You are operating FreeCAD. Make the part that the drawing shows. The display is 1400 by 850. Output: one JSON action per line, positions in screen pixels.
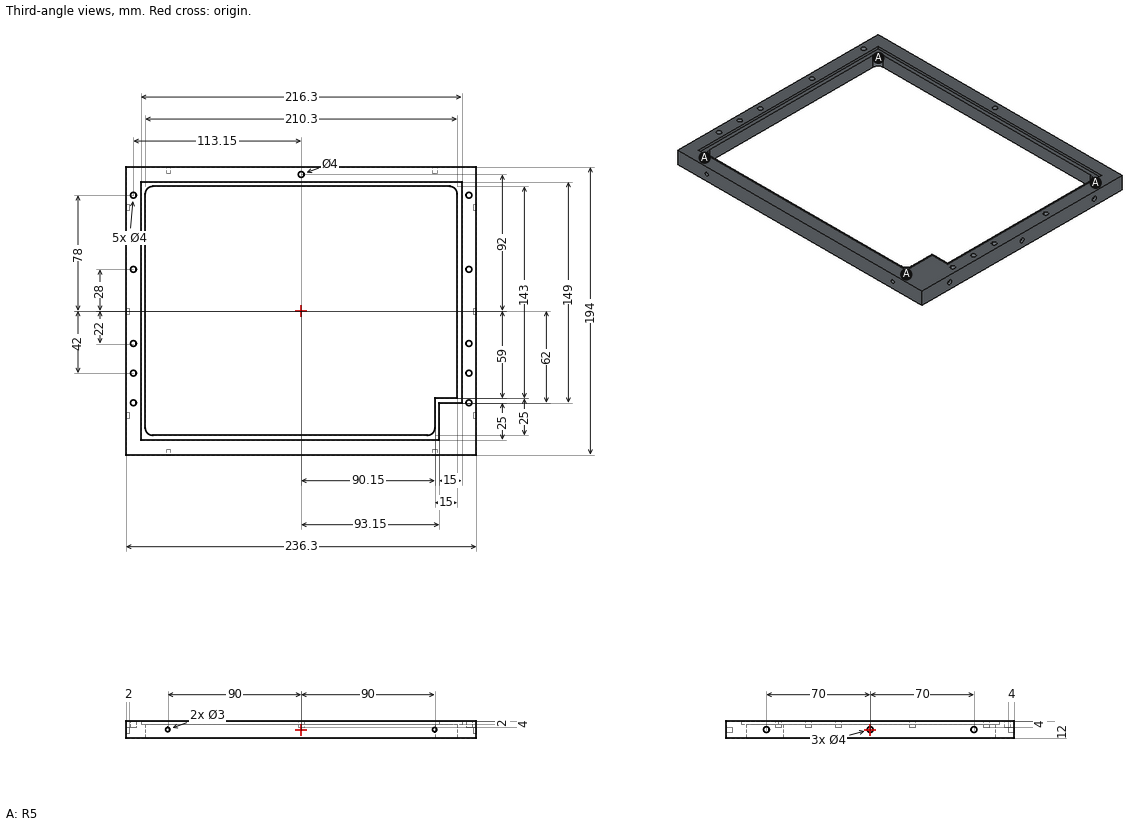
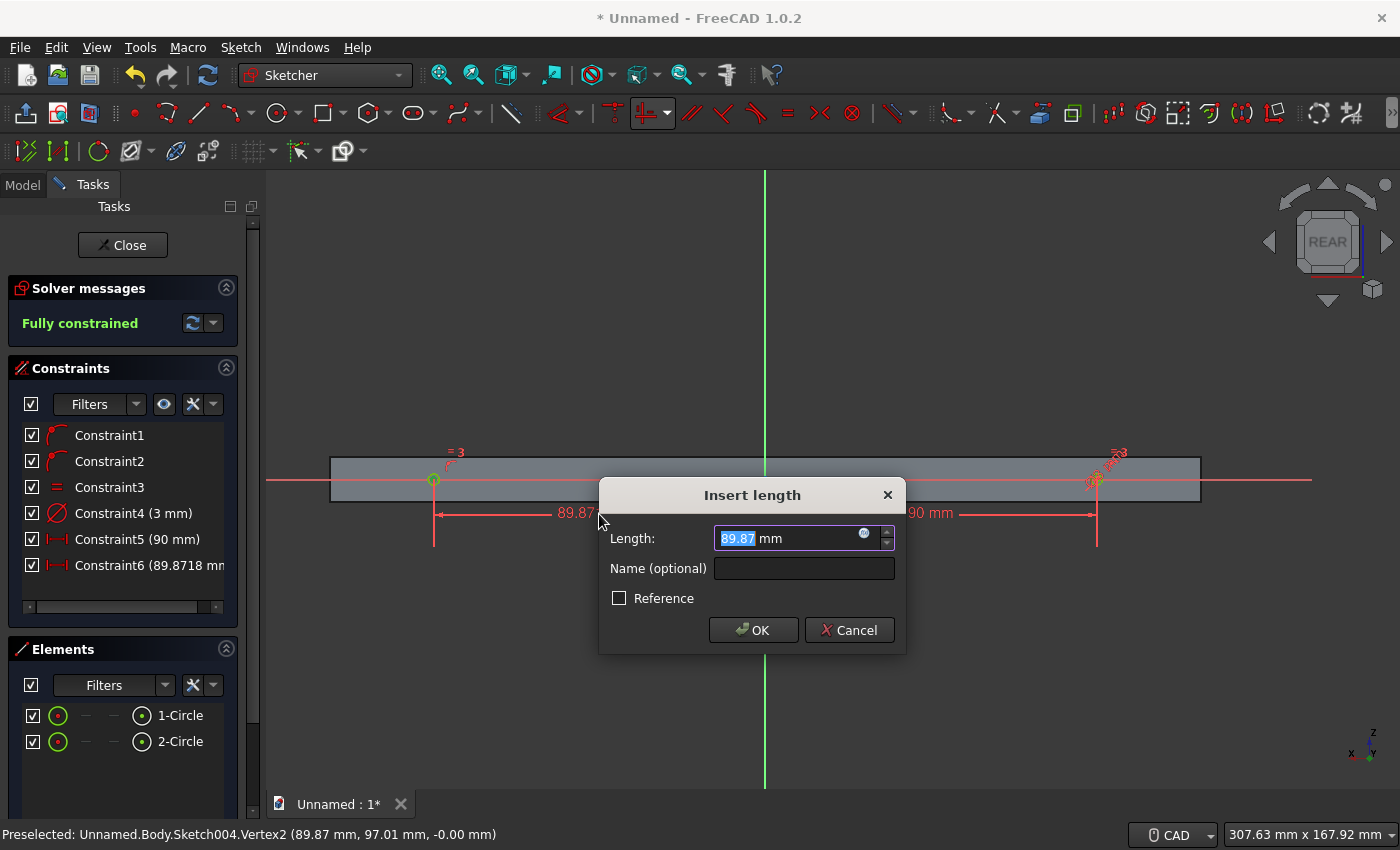
{"action": "type", "text": "90"}
{"action": "key", "text": "Return"}
{"action": "key", "text": "Escape"}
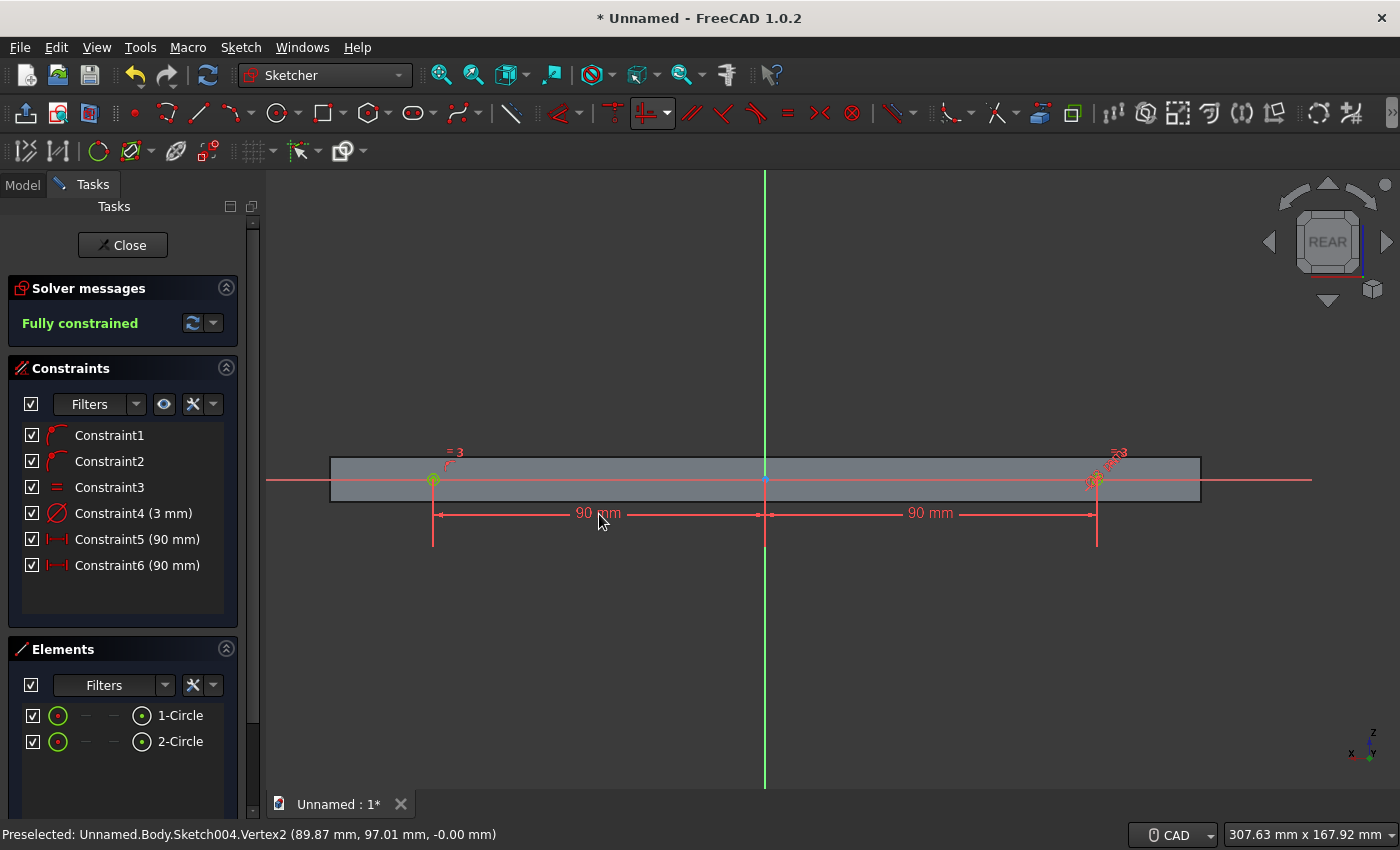
{"action": "left_click", "coordinate": [123, 245]}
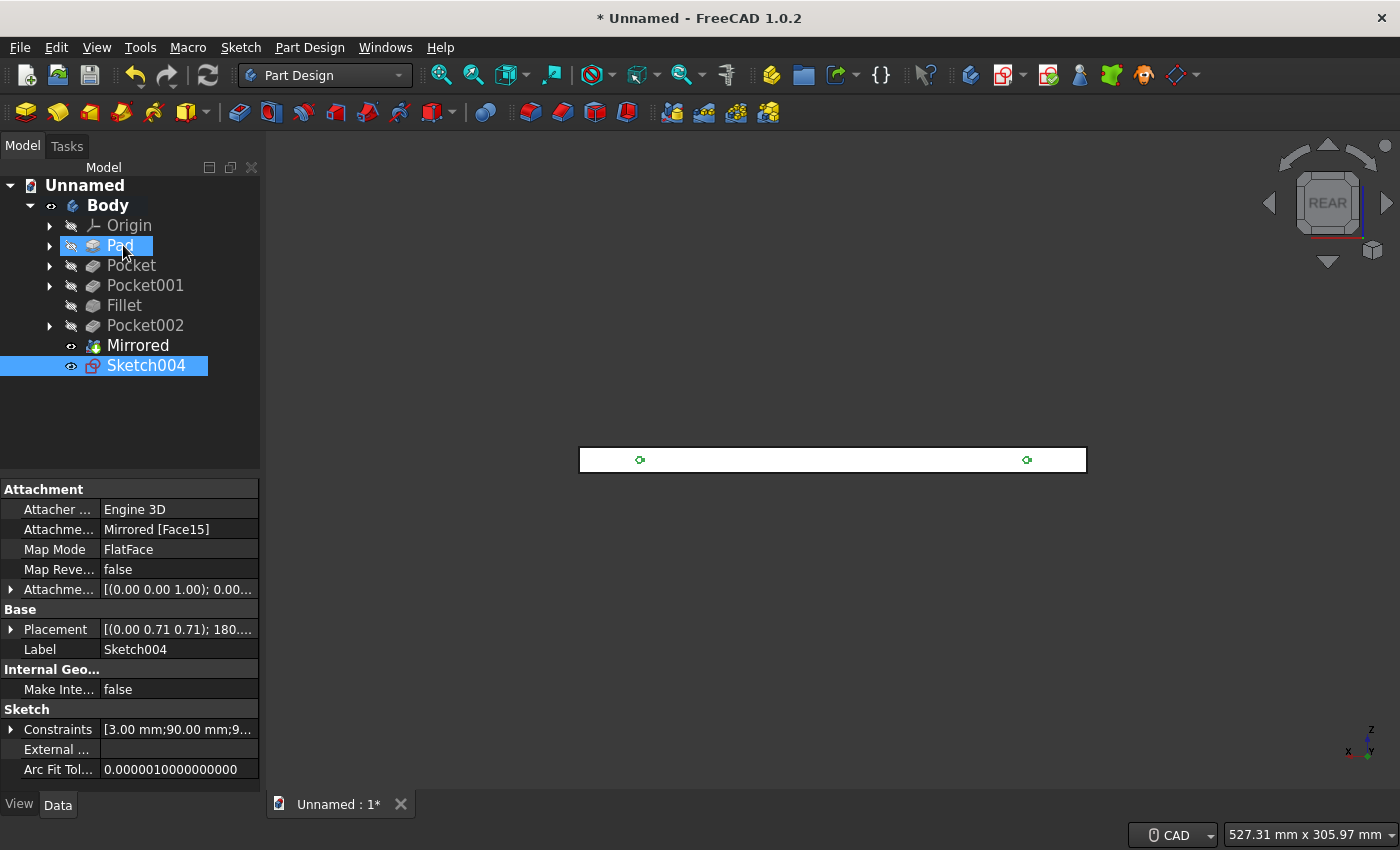
{"action": "left_click", "coordinate": [240, 112]}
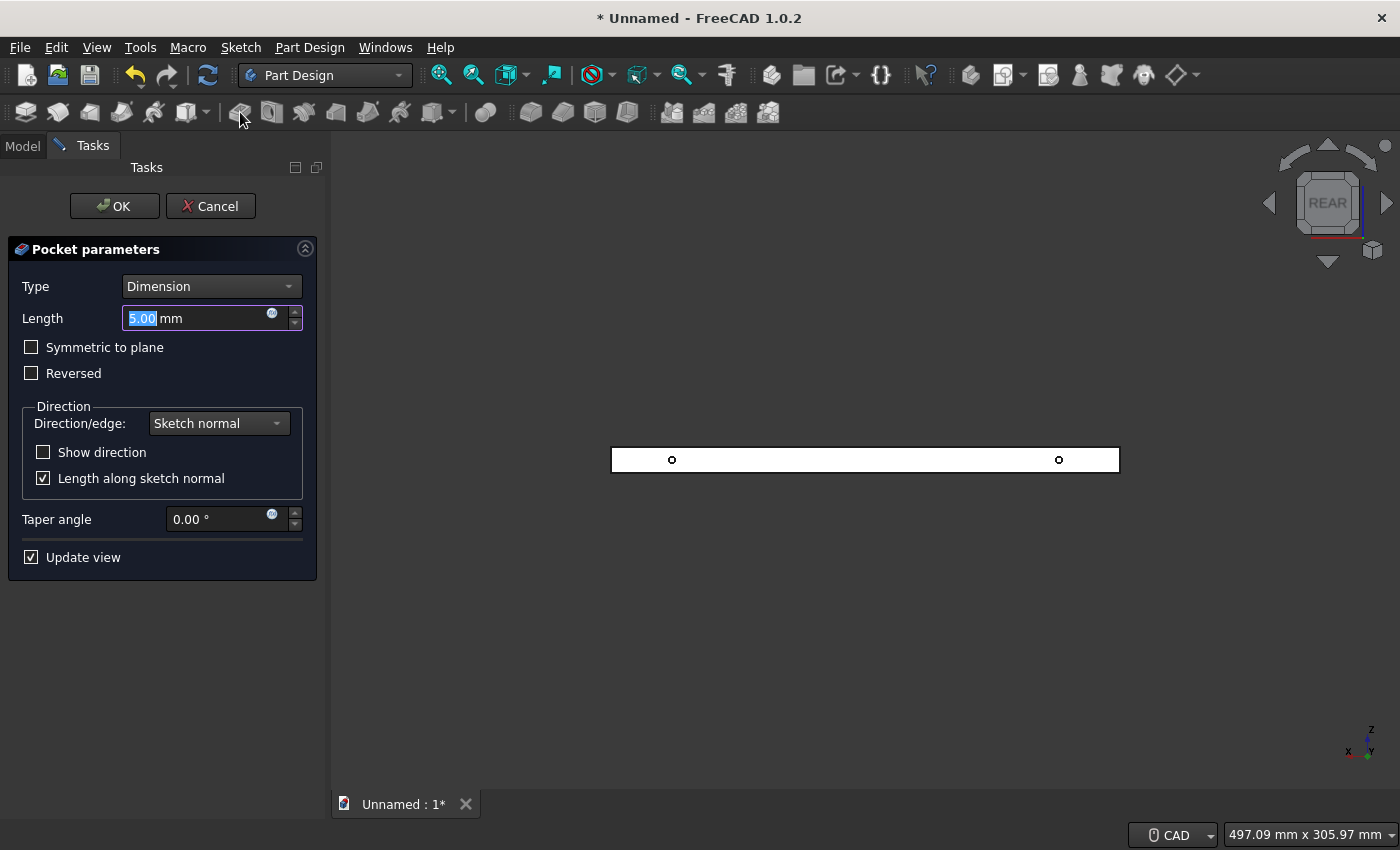
{"action": "type", "text": "4"}
{"action": "key", "text": "Tab"}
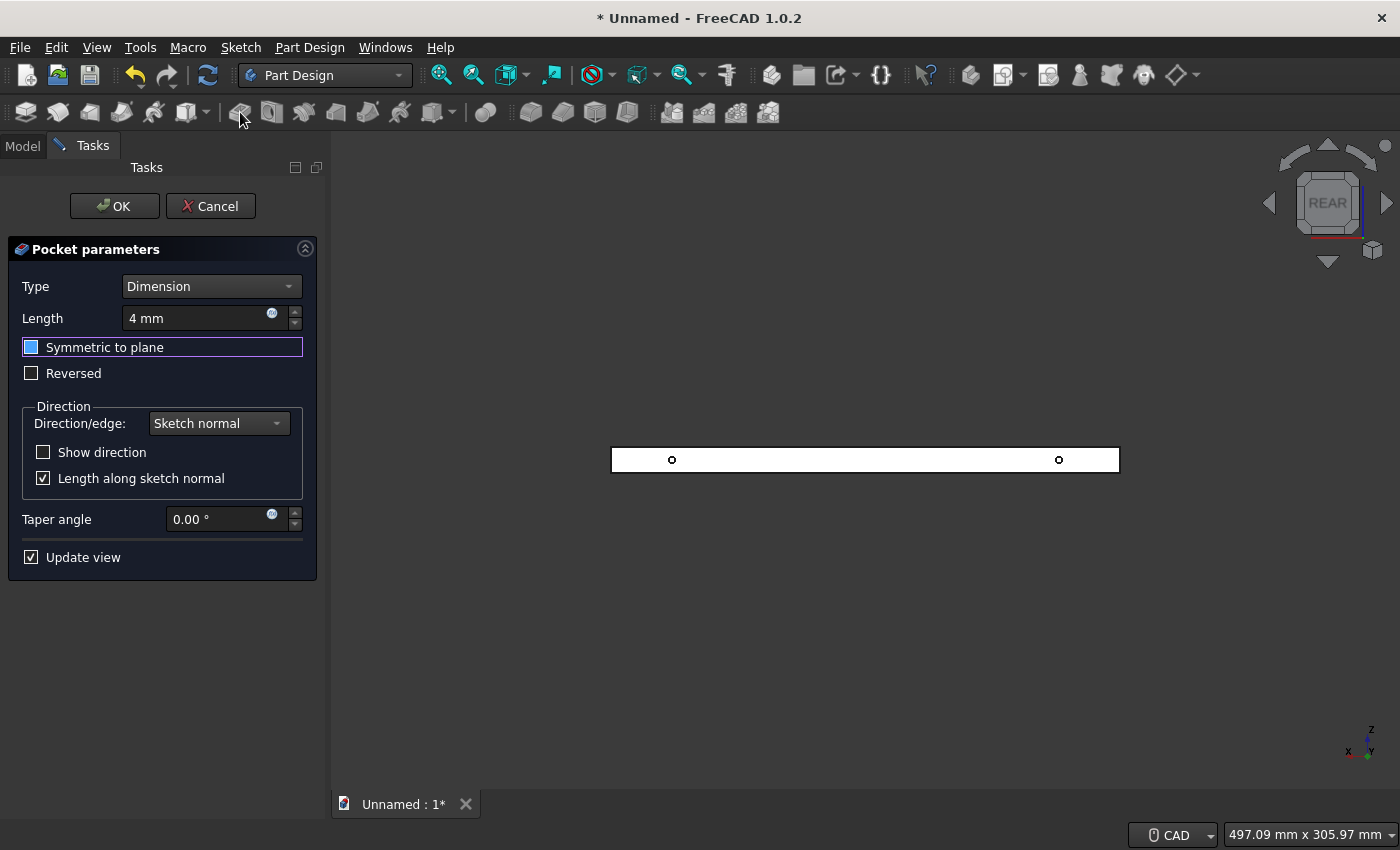
{"action": "left_click", "coordinate": [115, 206]}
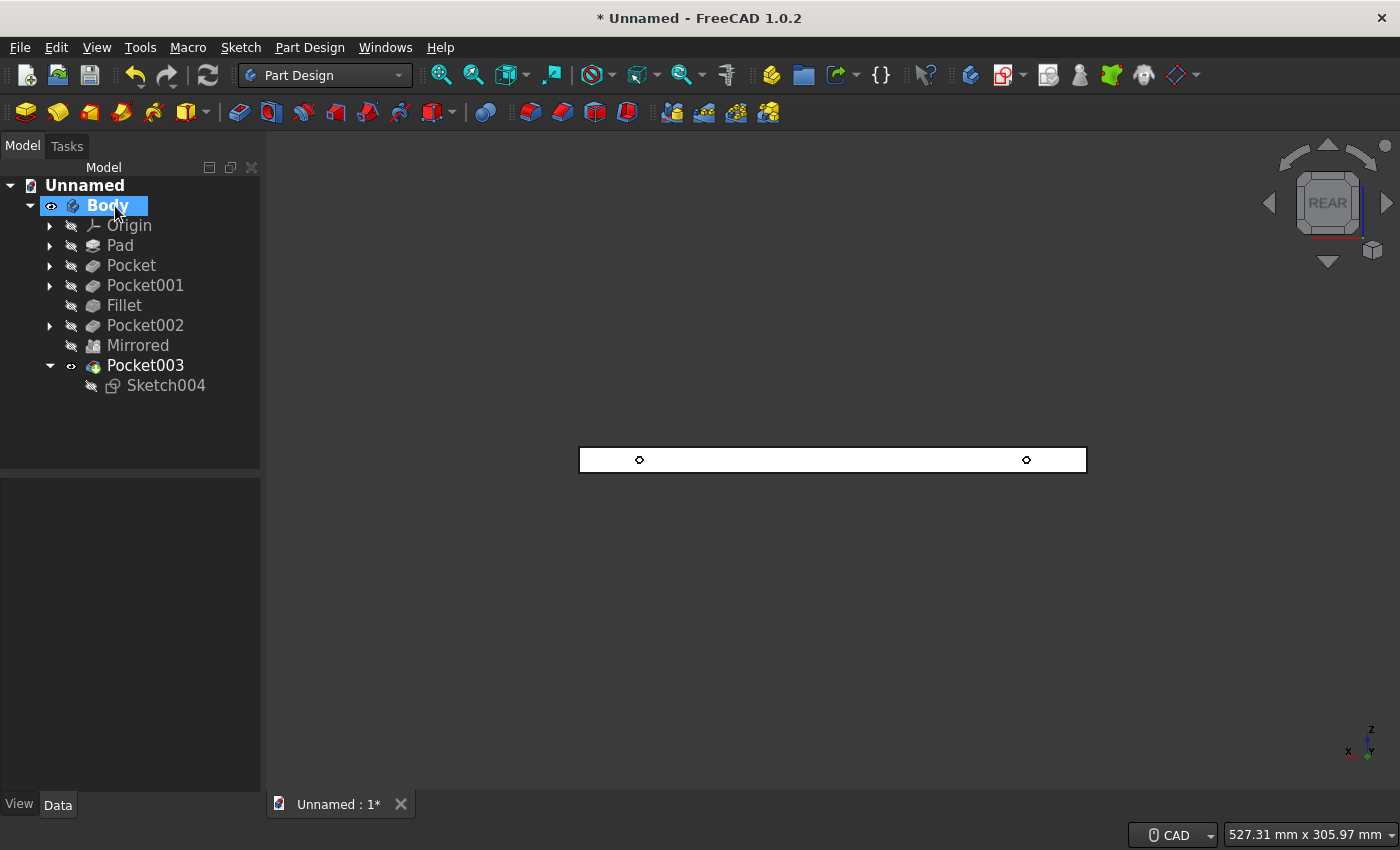
{"action": "left_click", "coordinate": [442, 76]}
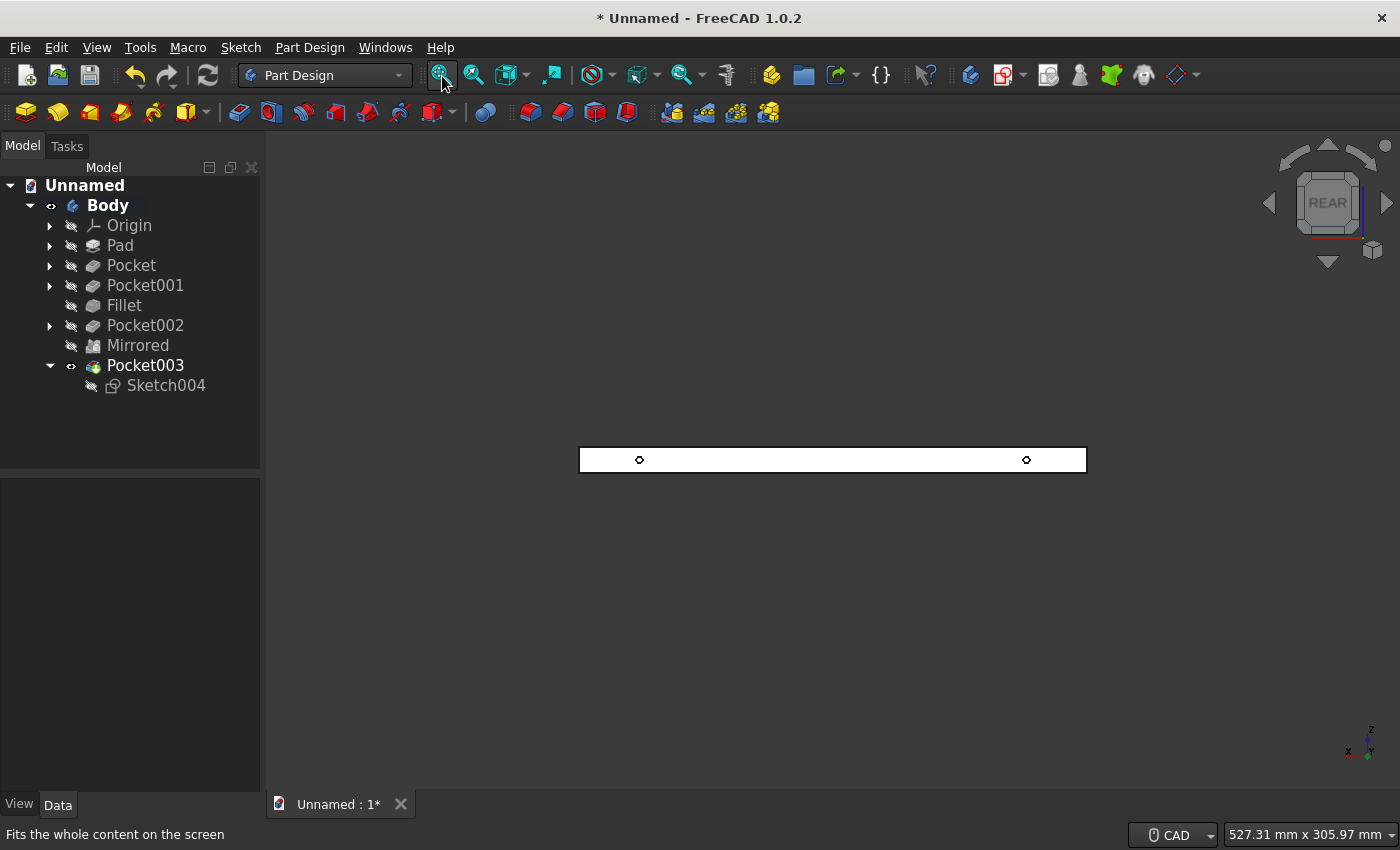
{"action": "left_click", "coordinate": [116, 366]}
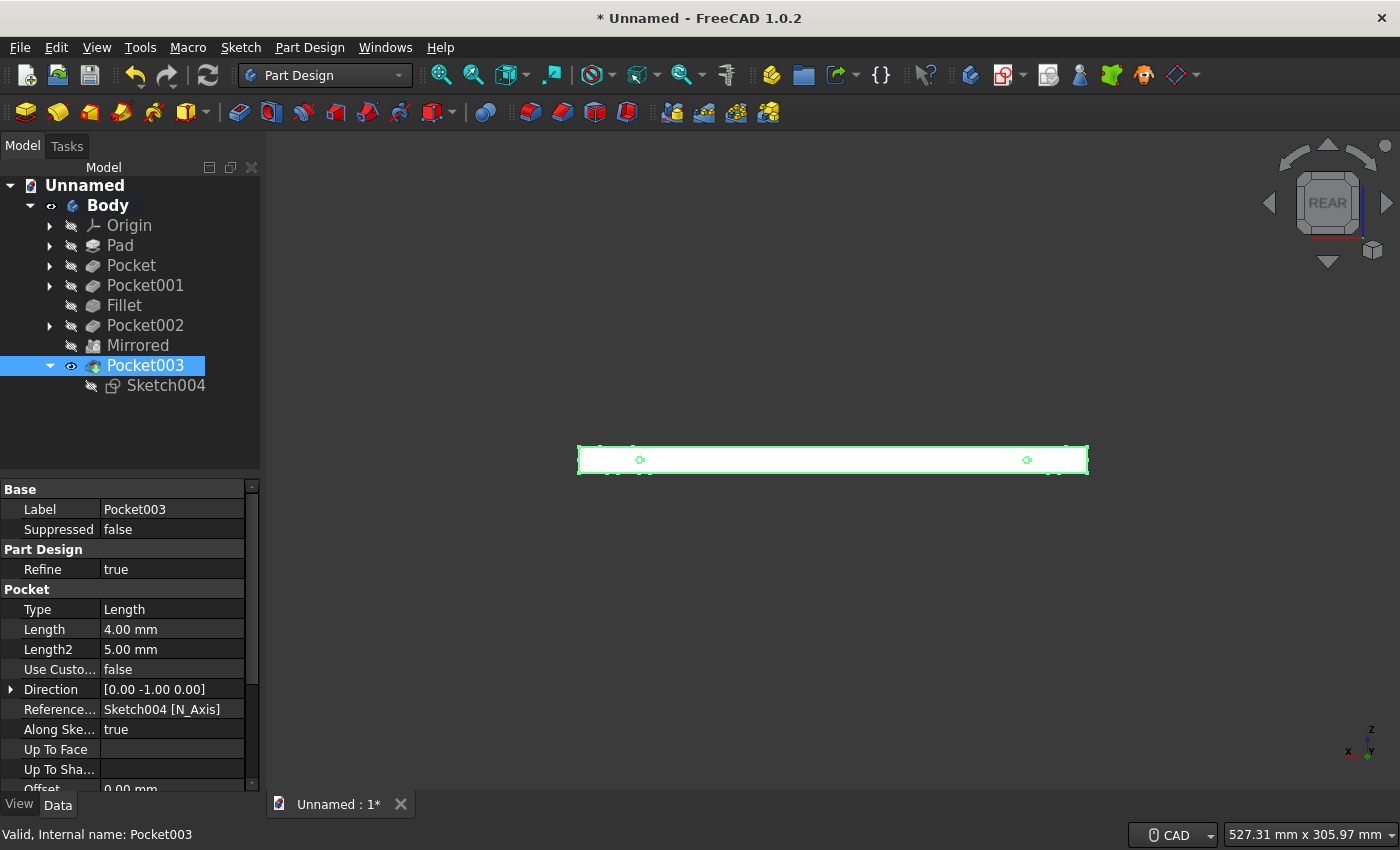
{"action": "left_click", "coordinate": [672, 112]}